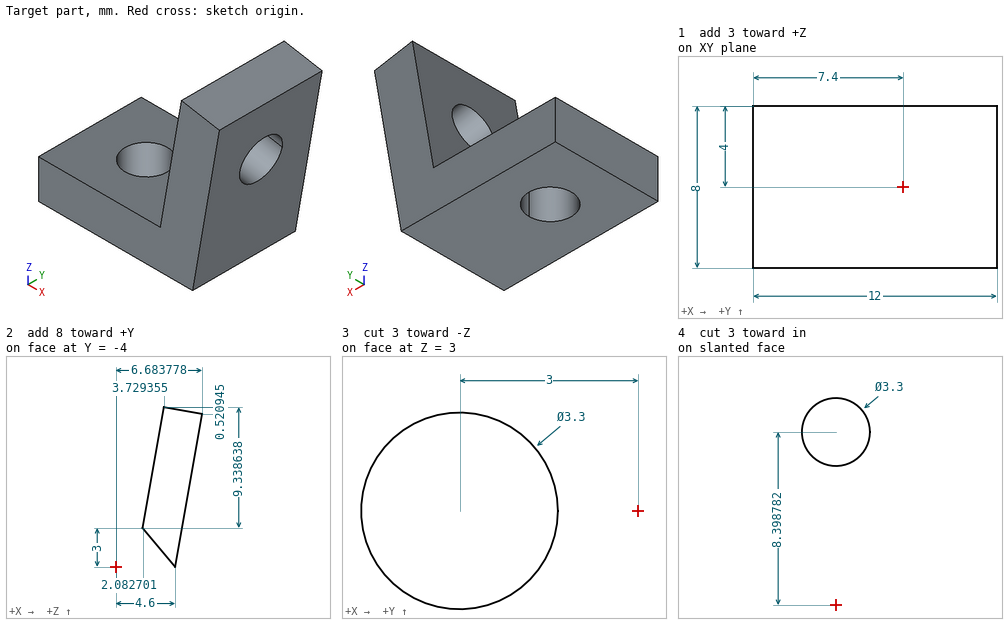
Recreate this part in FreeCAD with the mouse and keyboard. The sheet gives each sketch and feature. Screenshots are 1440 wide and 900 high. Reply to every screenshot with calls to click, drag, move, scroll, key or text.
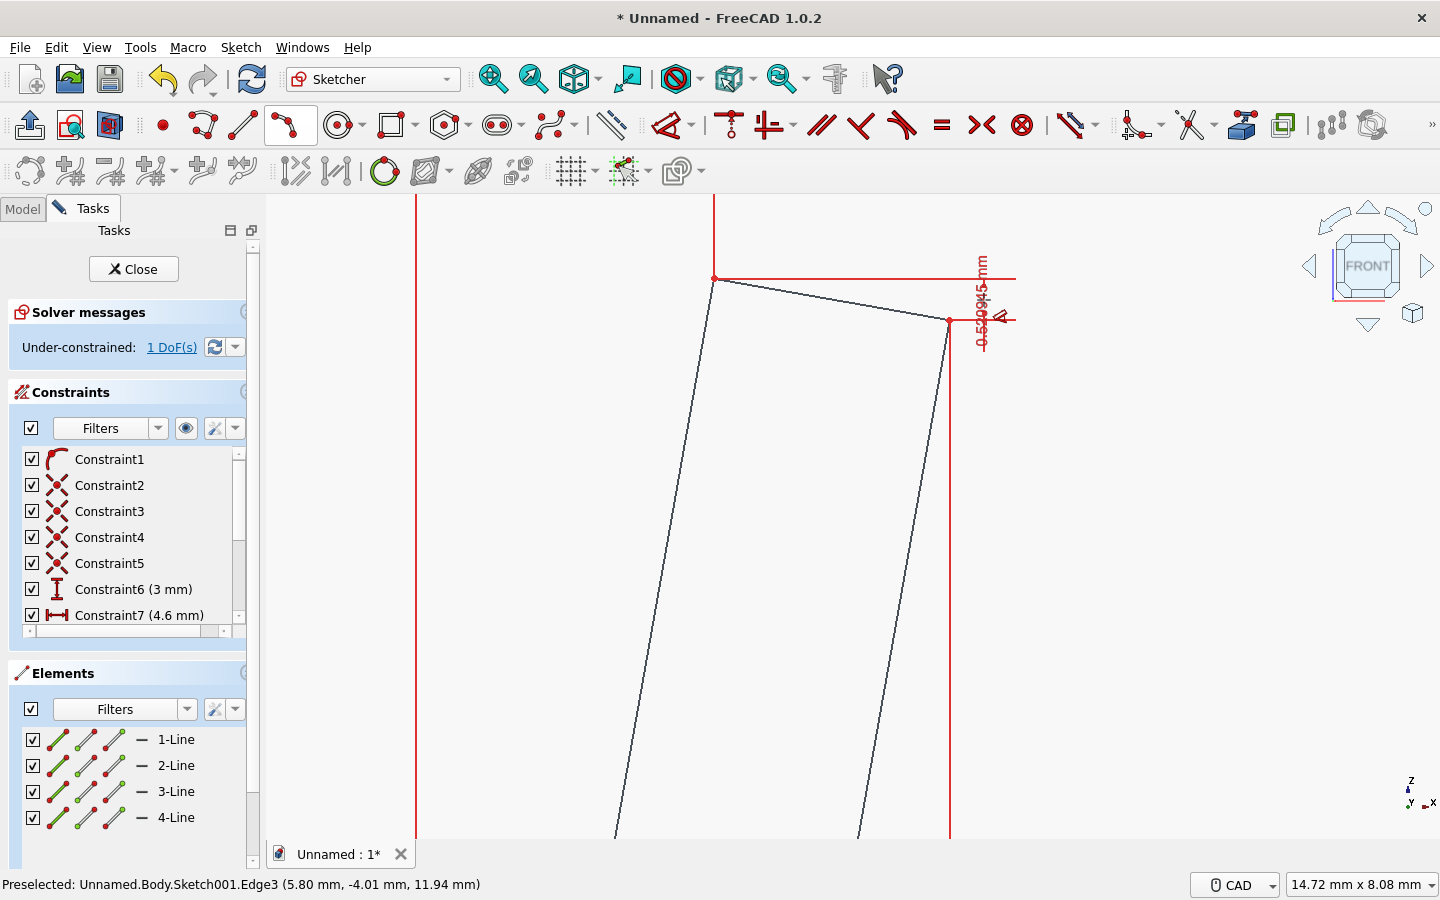
click(675, 501)
click(549, 545)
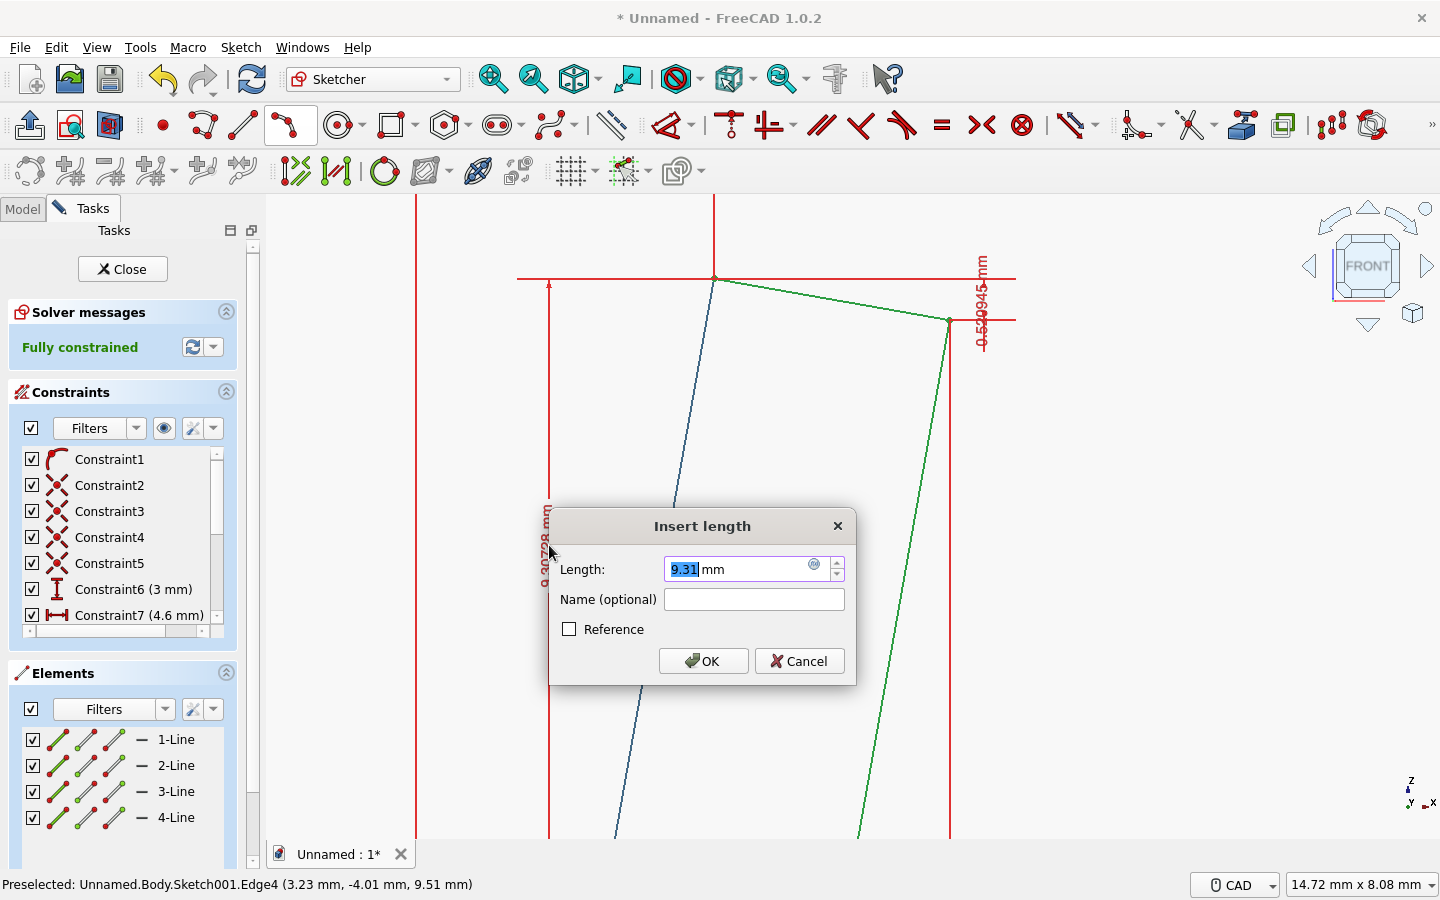
text(9.338638)
key(Return)
key(Escape)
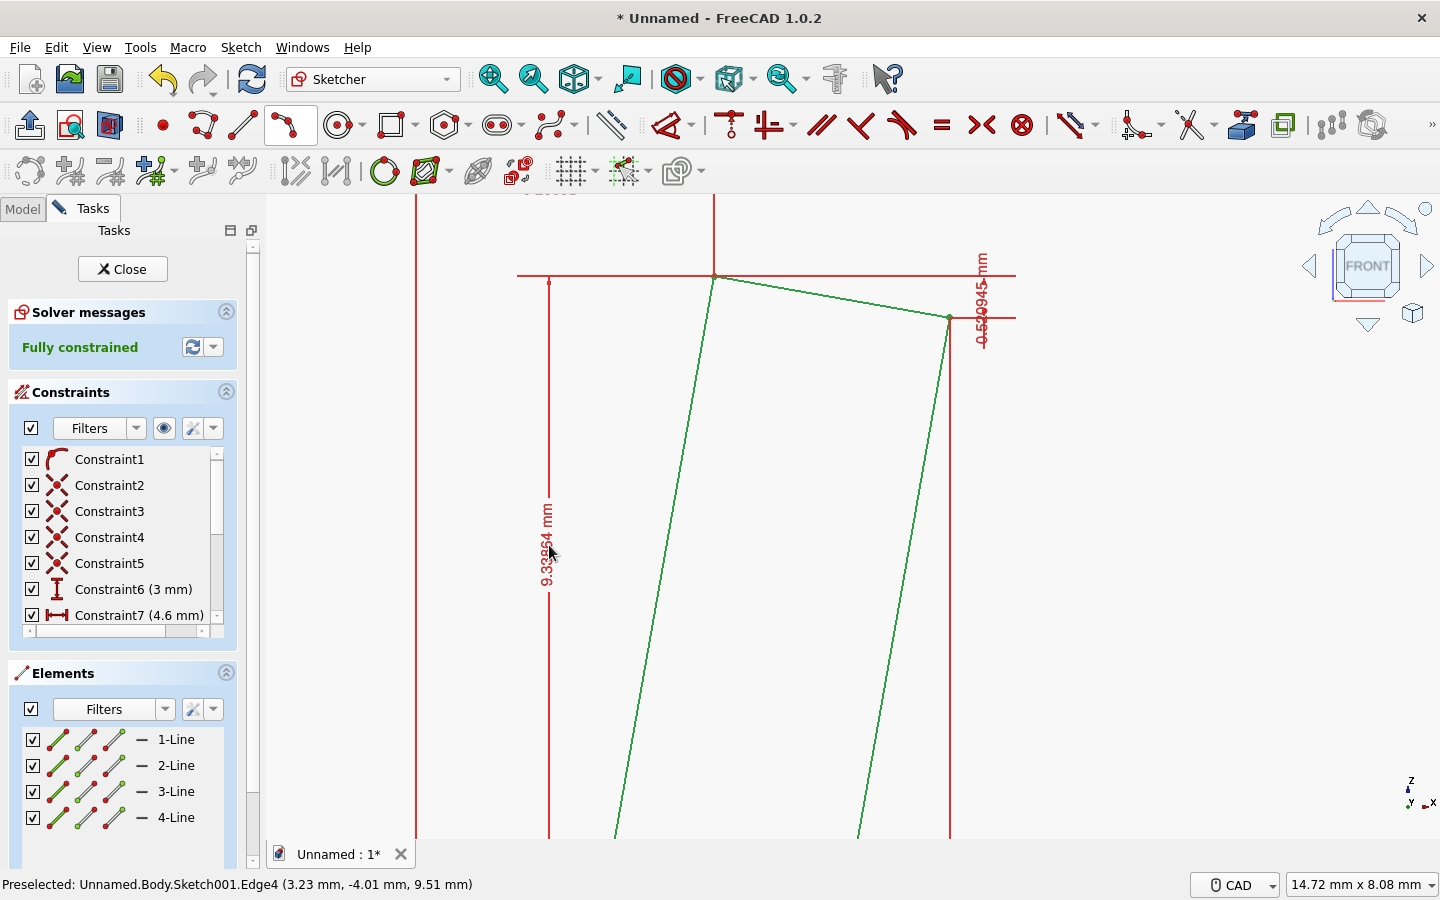
click(123, 269)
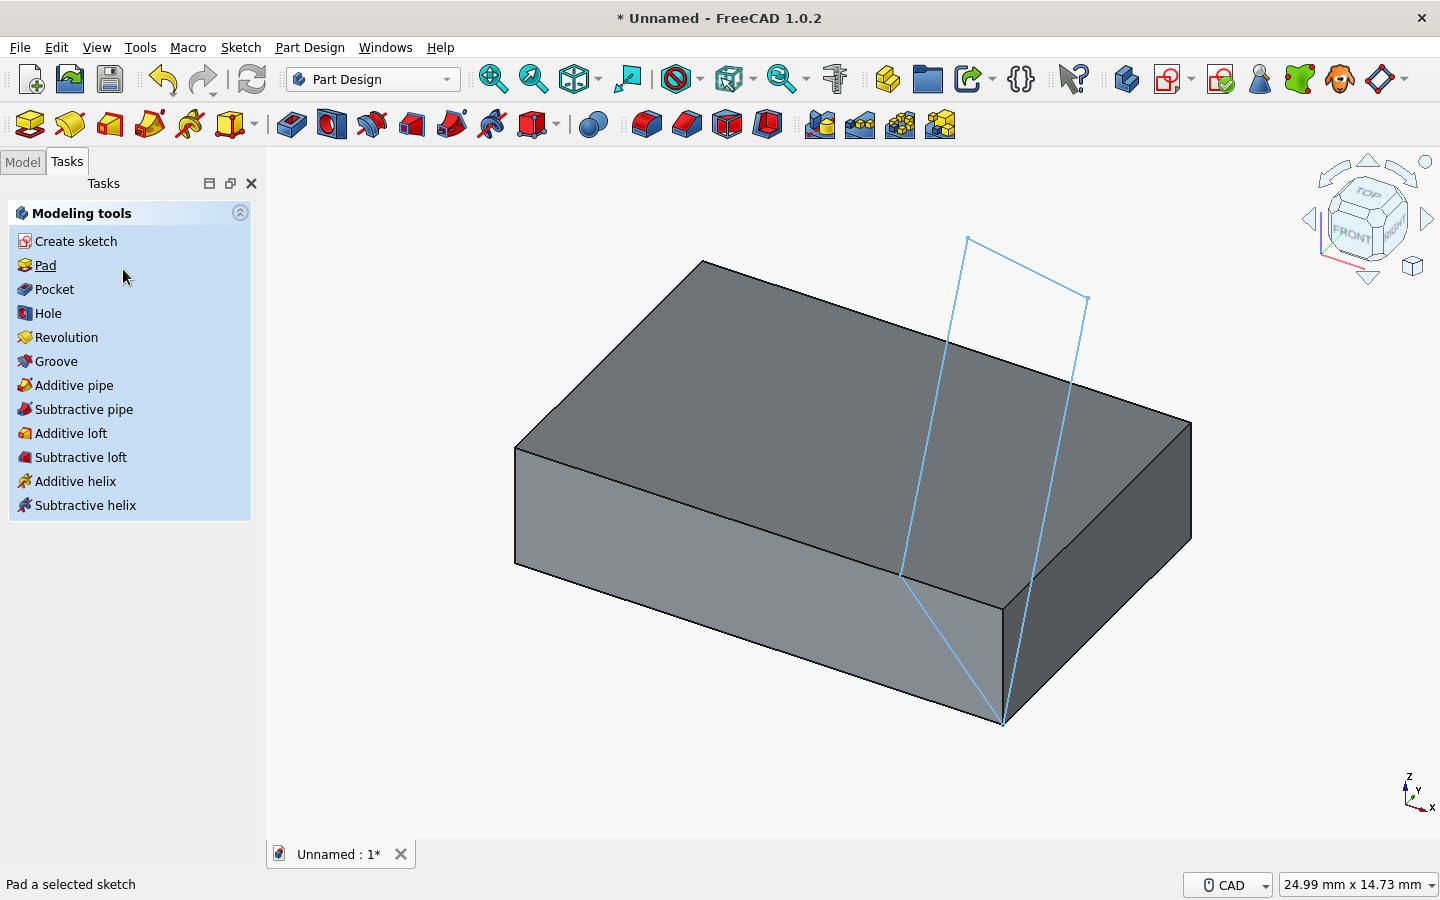
click(30, 124)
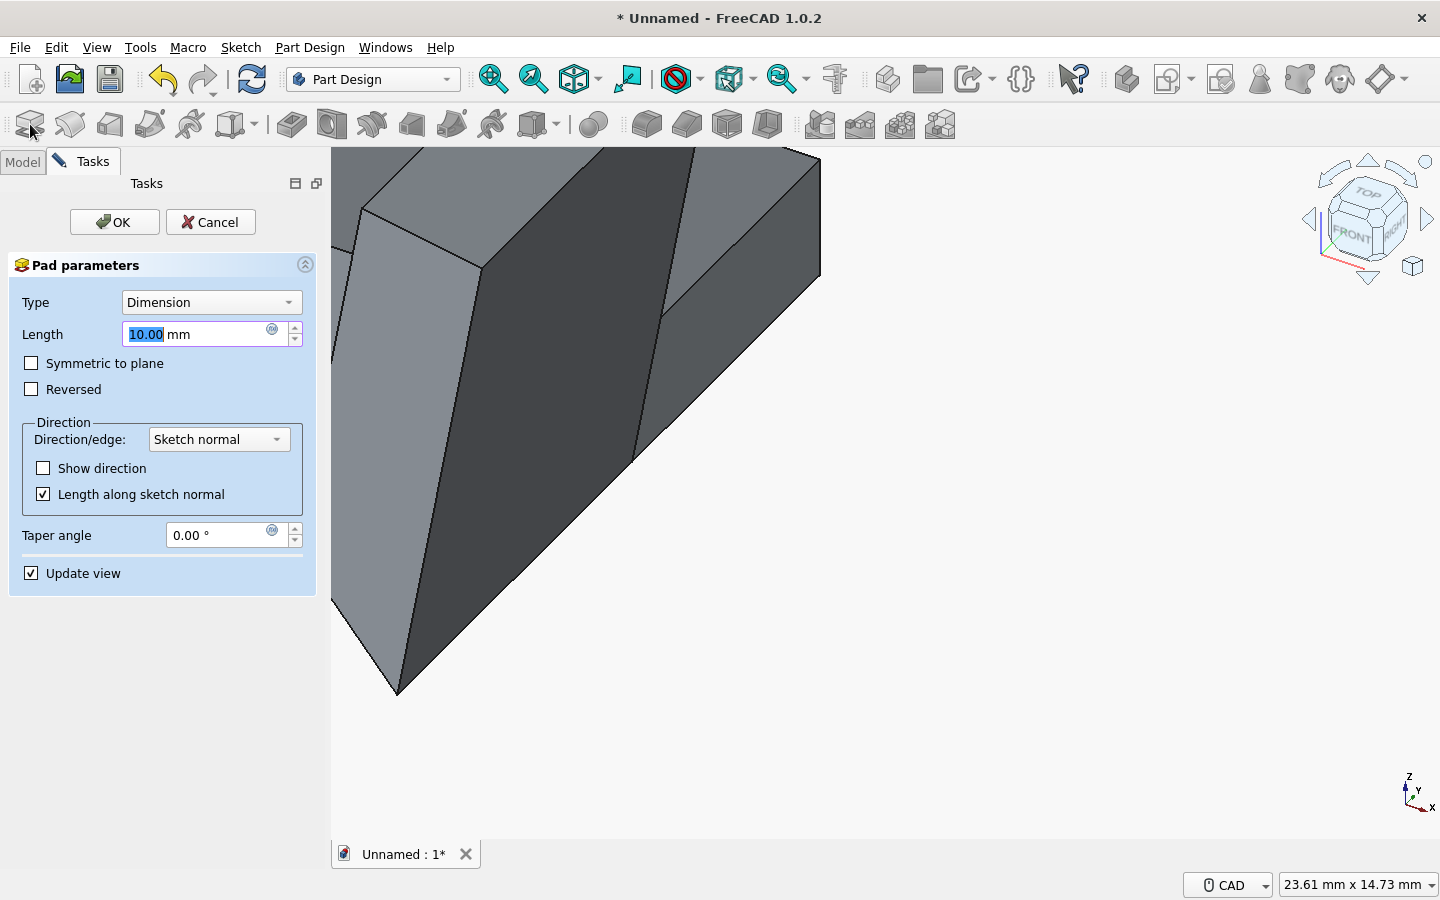
text(8)
key(Tab)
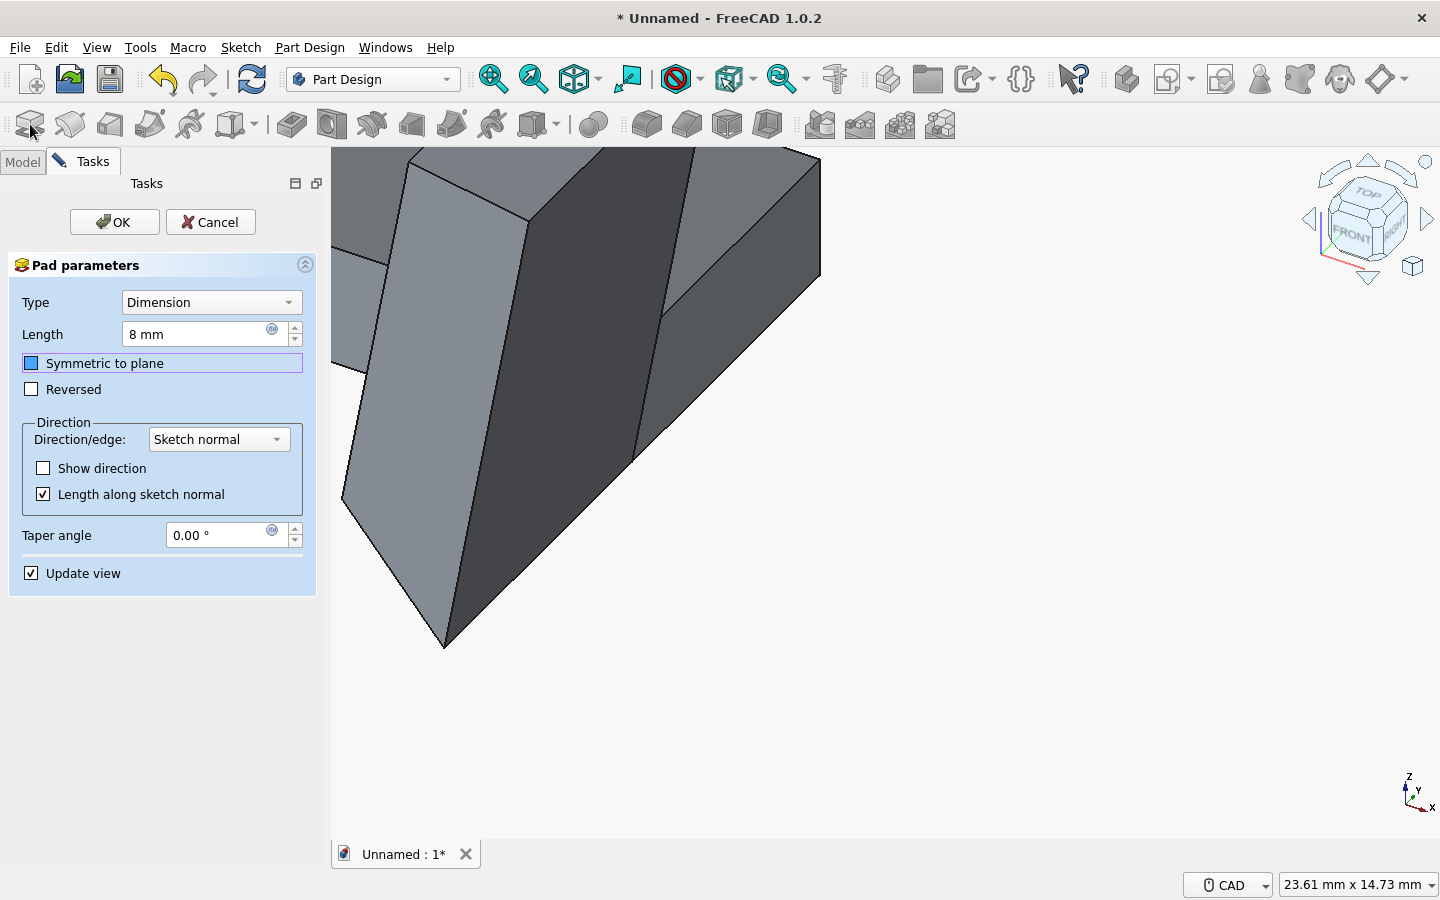
click(30, 389)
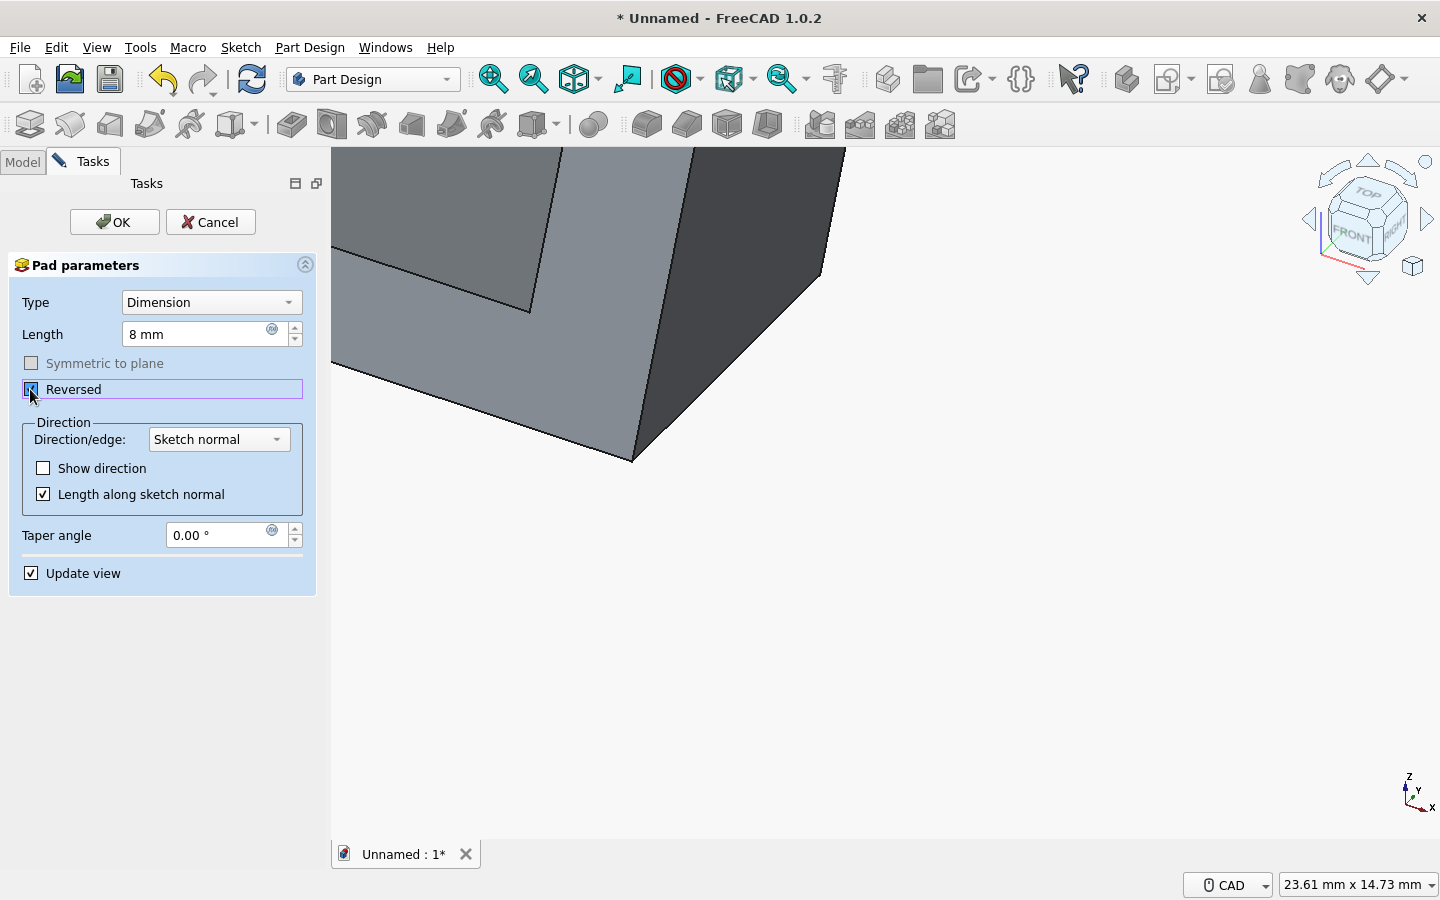
click(115, 222)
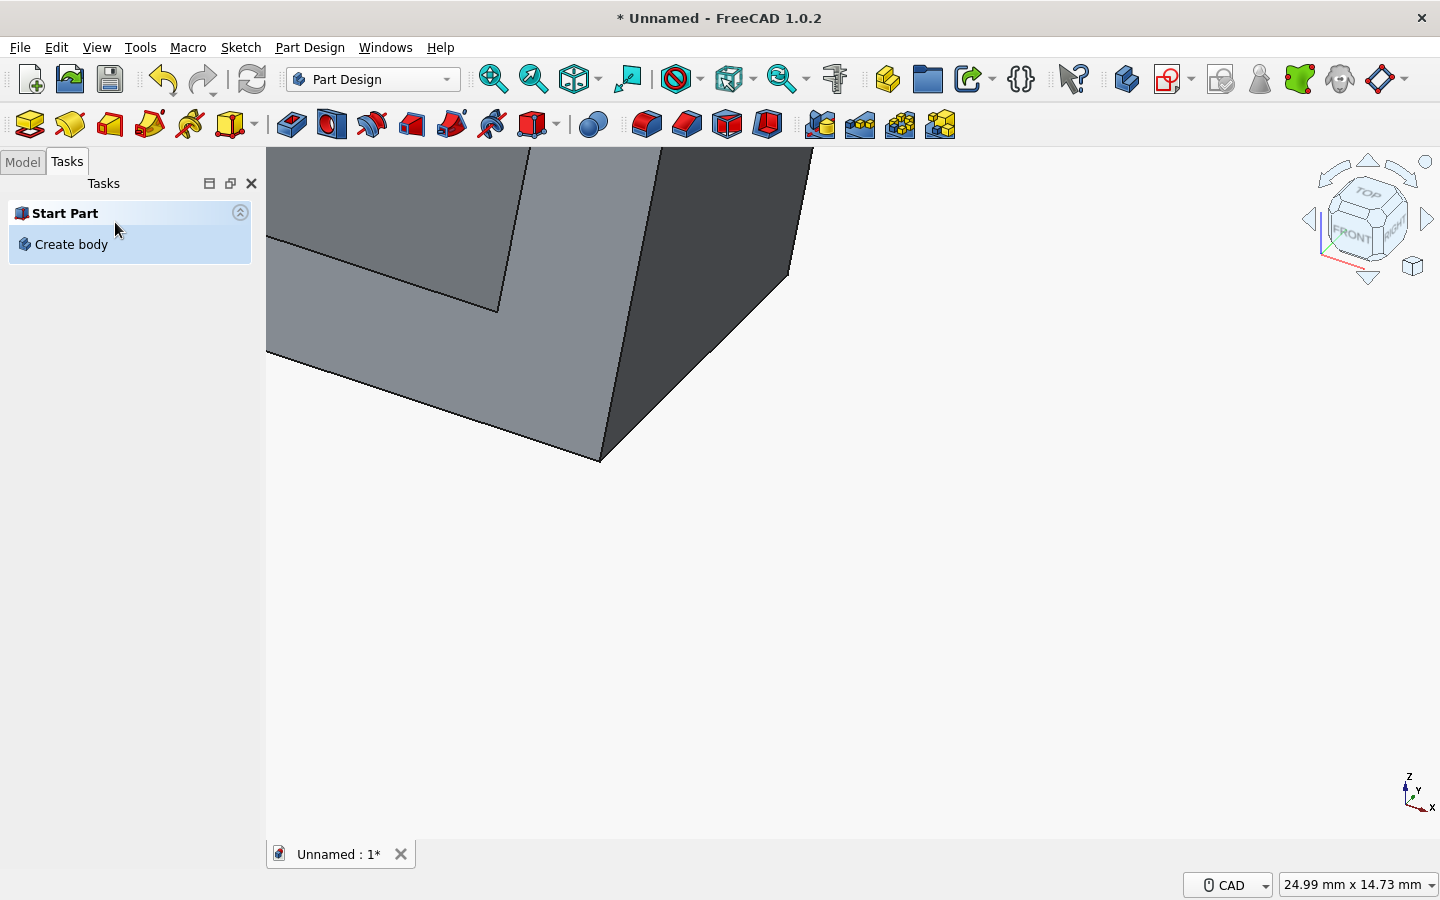
click(494, 80)